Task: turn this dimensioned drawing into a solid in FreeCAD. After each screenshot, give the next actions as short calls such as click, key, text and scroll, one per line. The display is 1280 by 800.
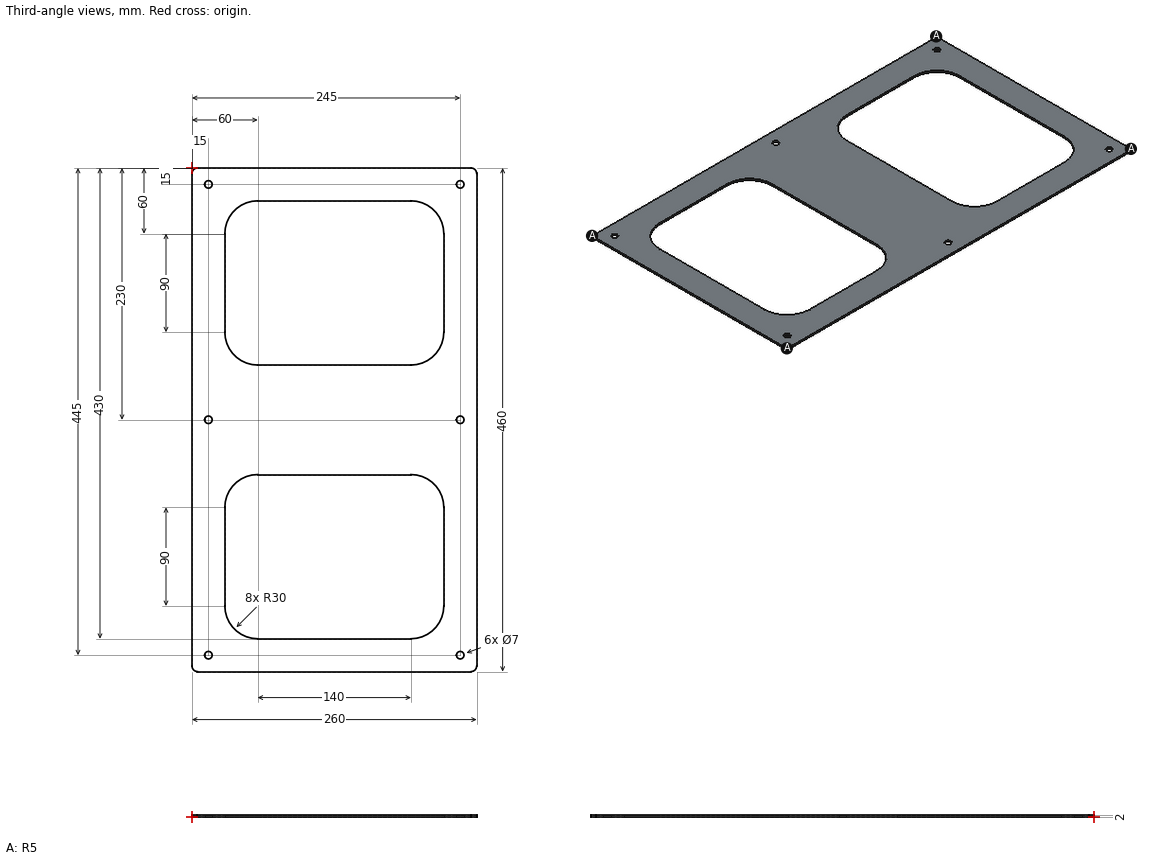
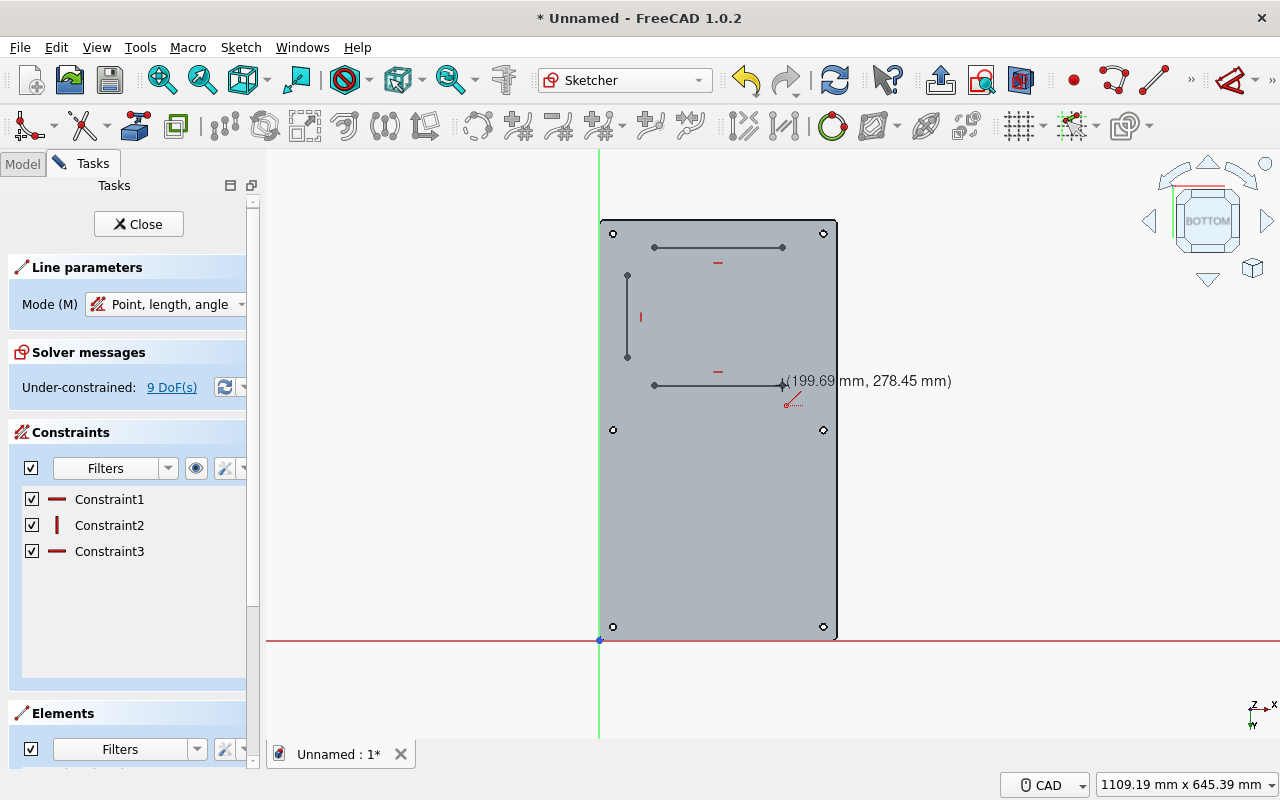
click(810, 357)
click(810, 275)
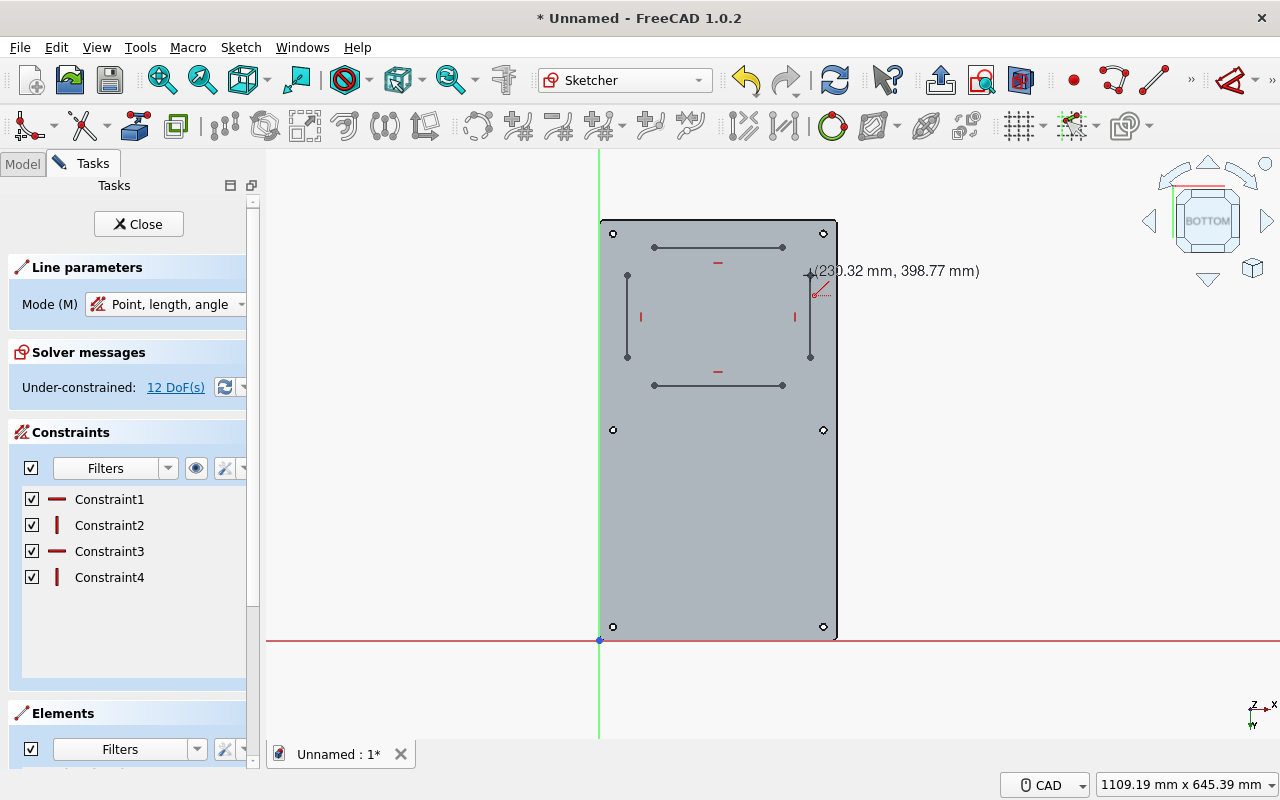
key(g)
key(3)
key(a)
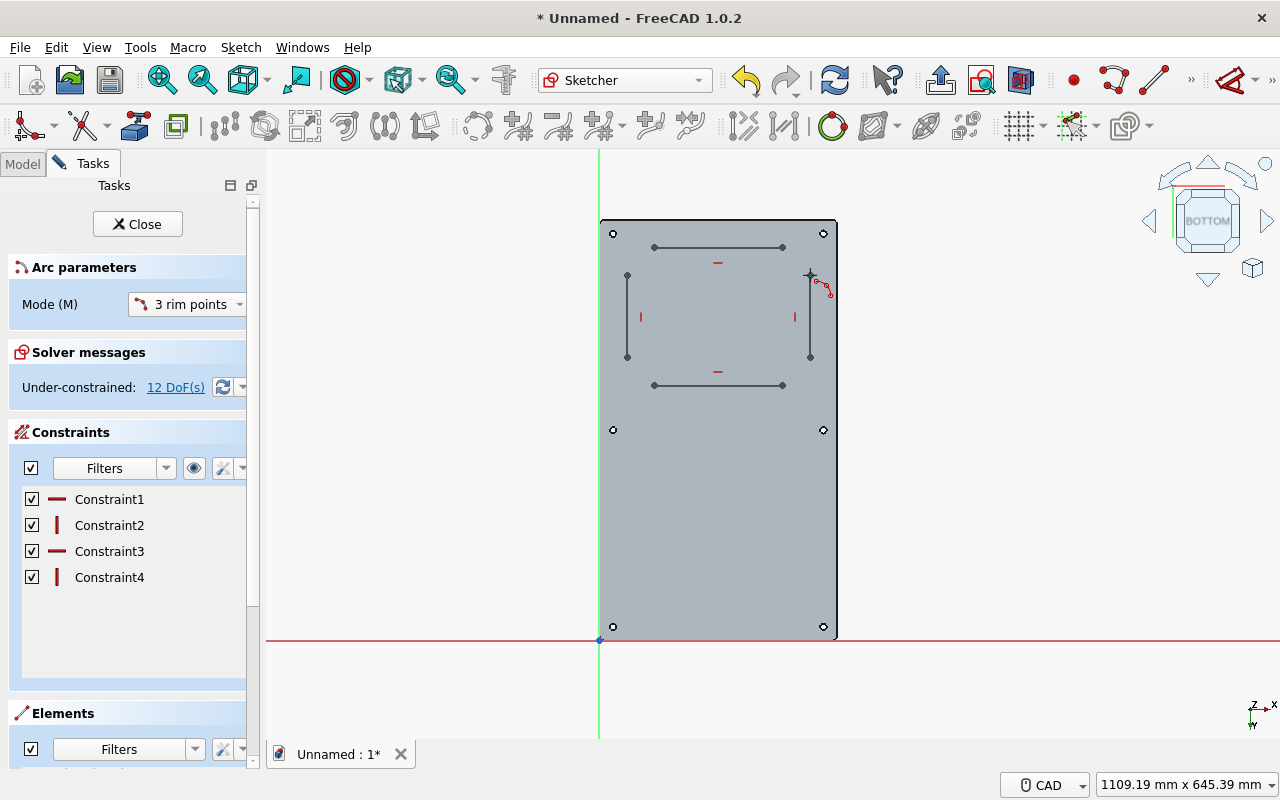
click(654, 248)
click(627, 276)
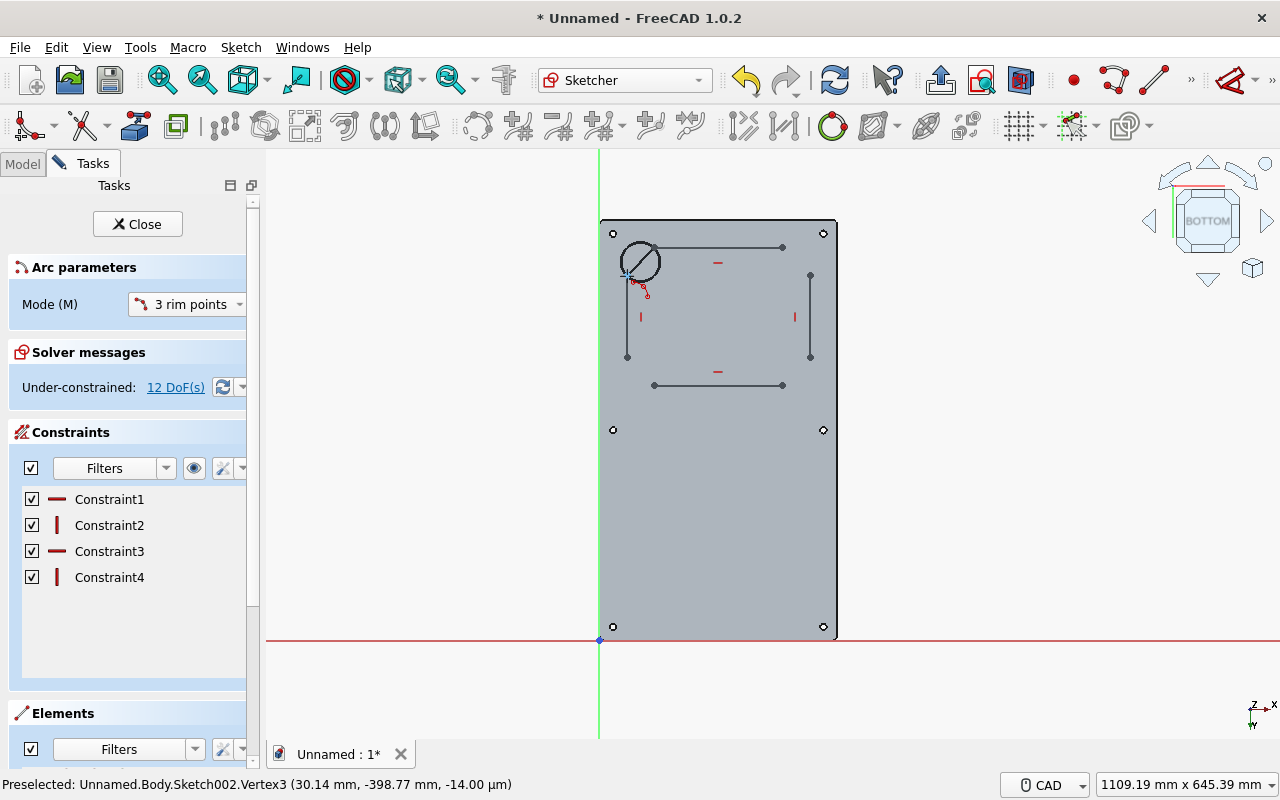
scroll(635, 255, up, 4)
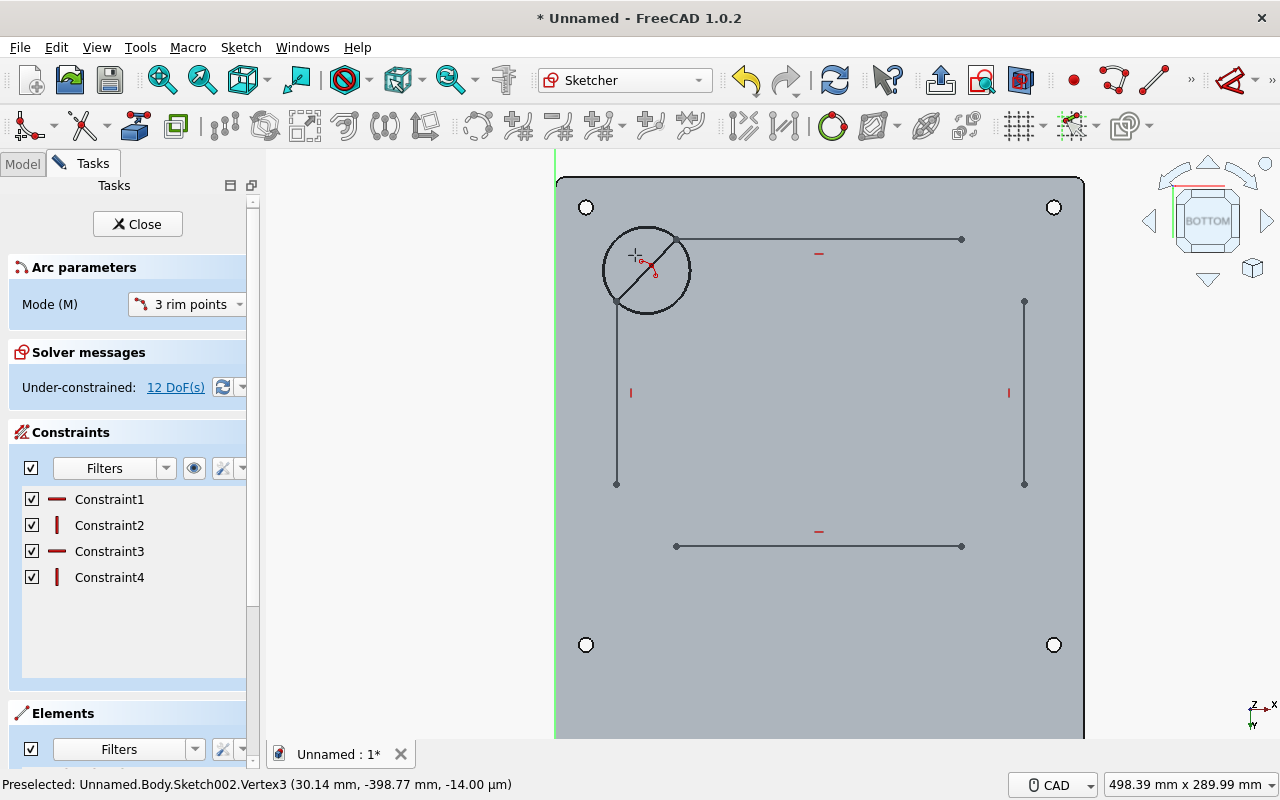
click(634, 256)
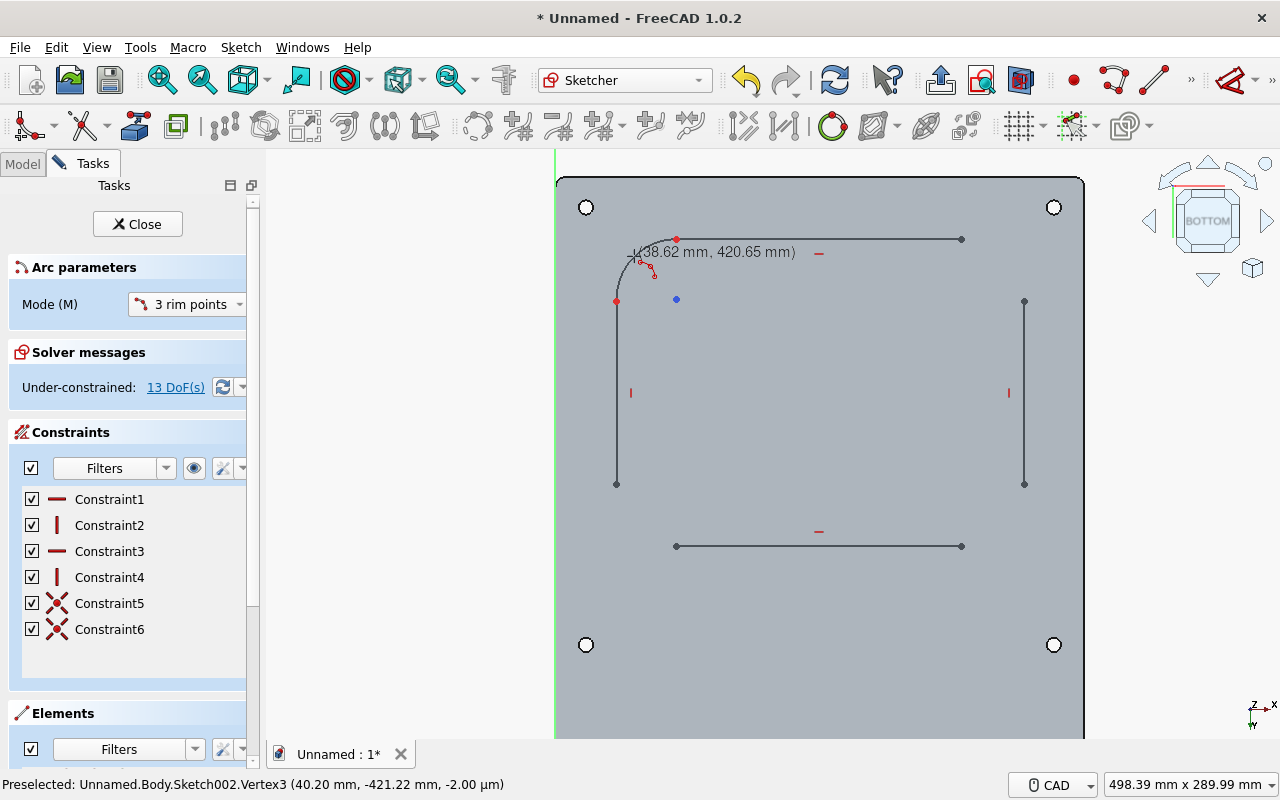
click(617, 484)
click(677, 546)
click(634, 525)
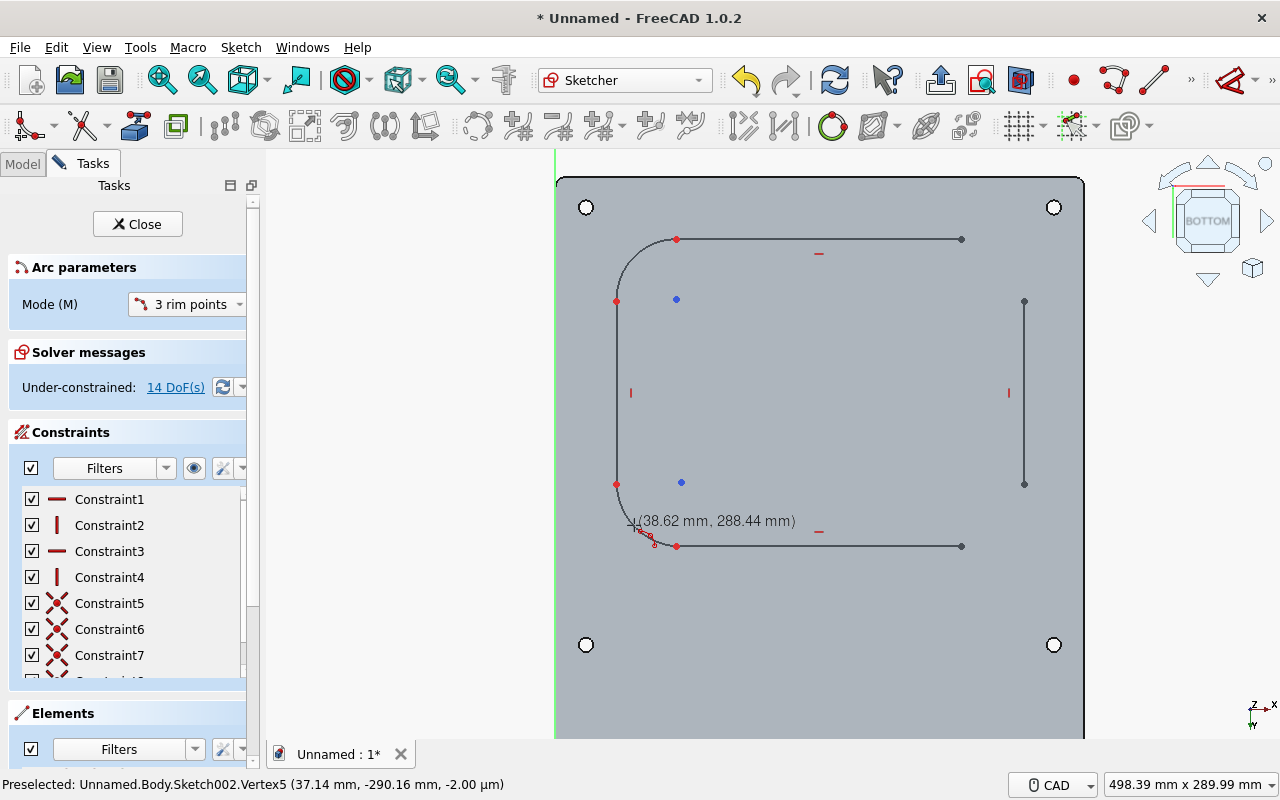
click(962, 546)
click(1024, 484)
click(1006, 525)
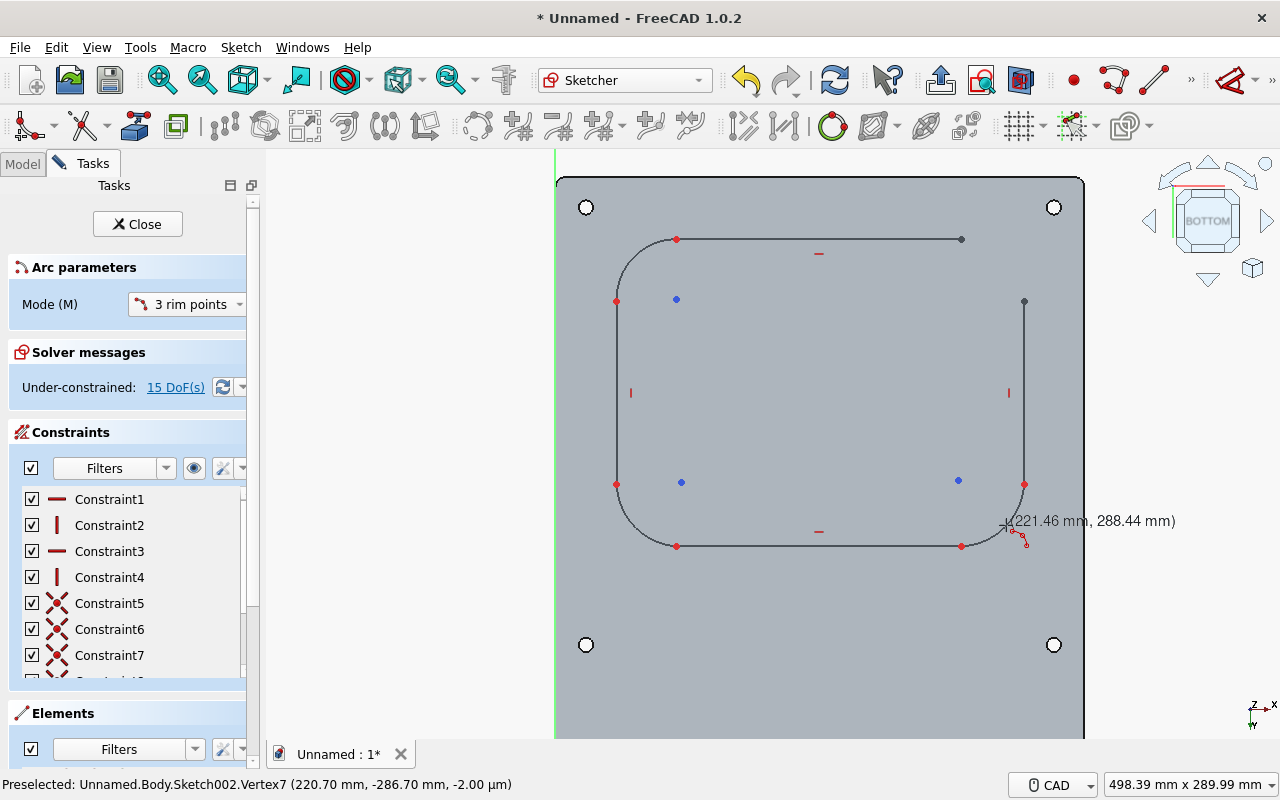
click(1024, 302)
click(962, 239)
click(1006, 256)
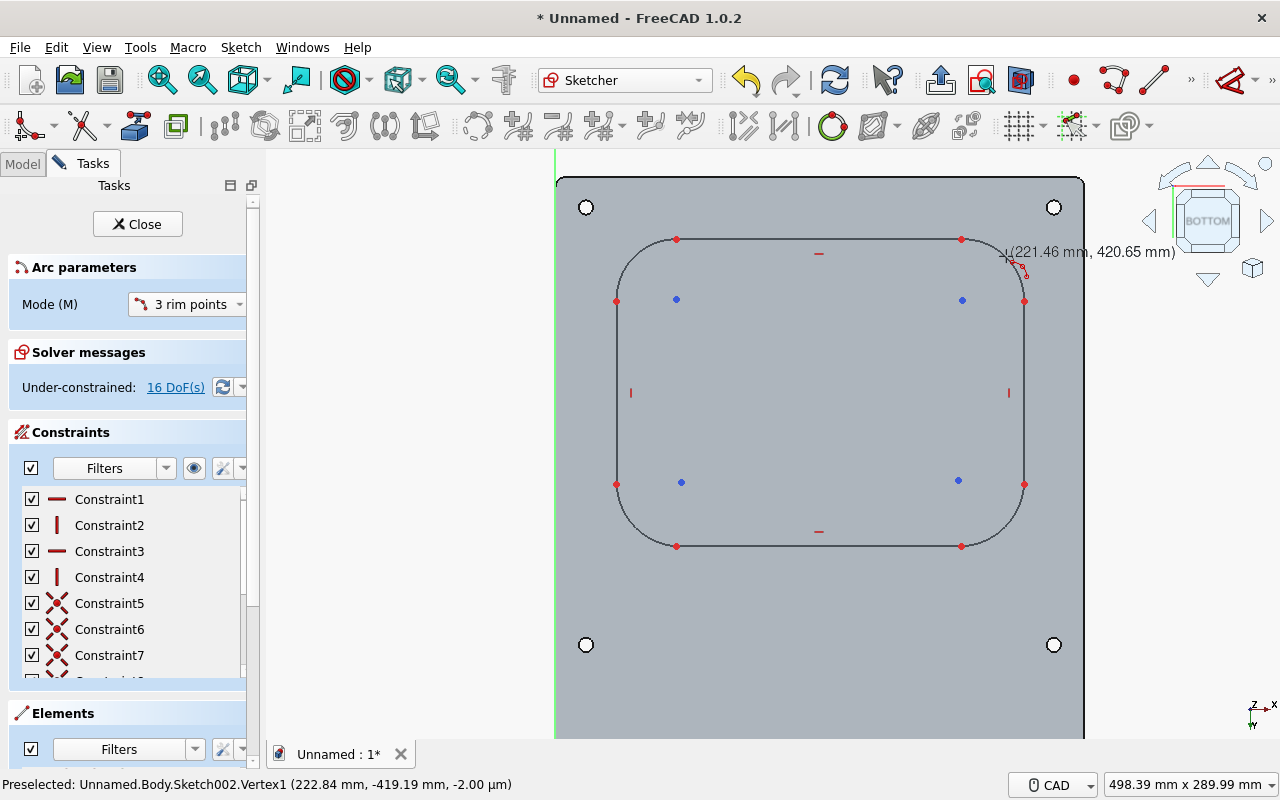
click(1154, 80)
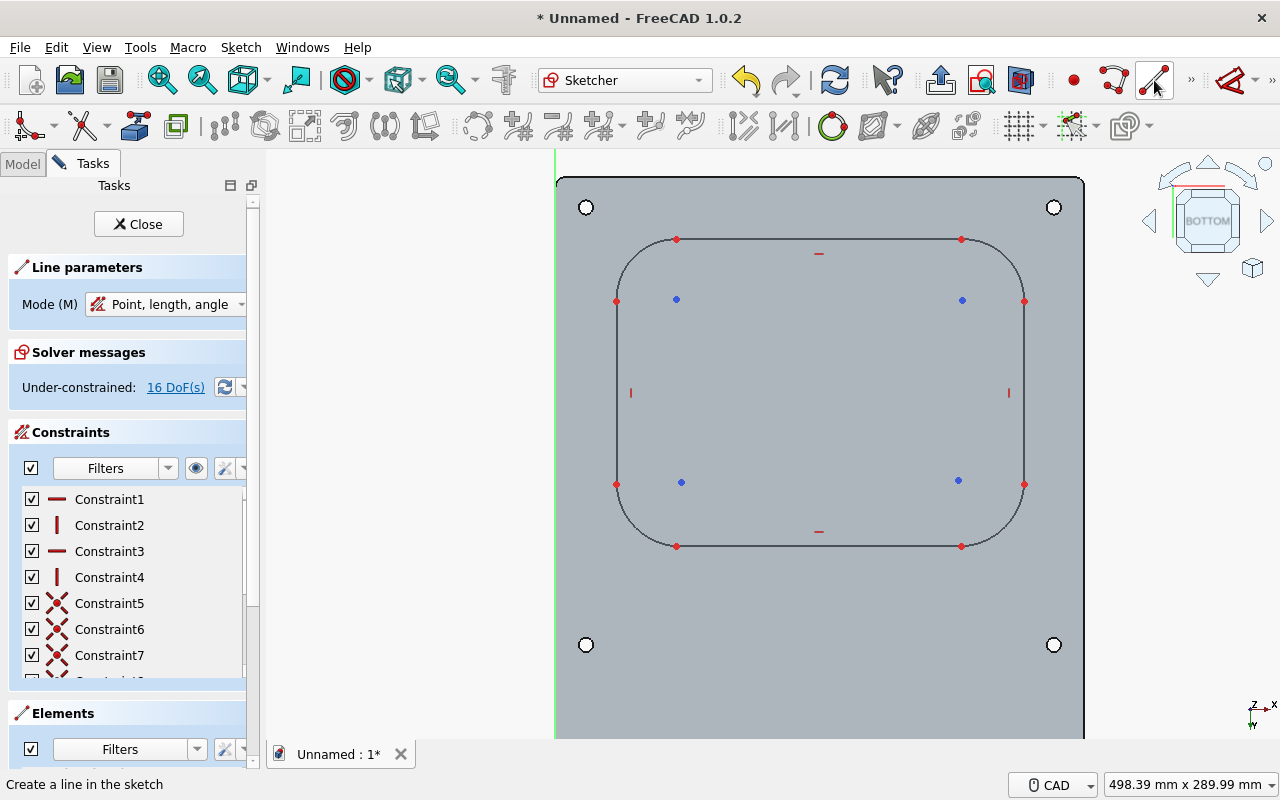
scroll(635, 255, down, 4)